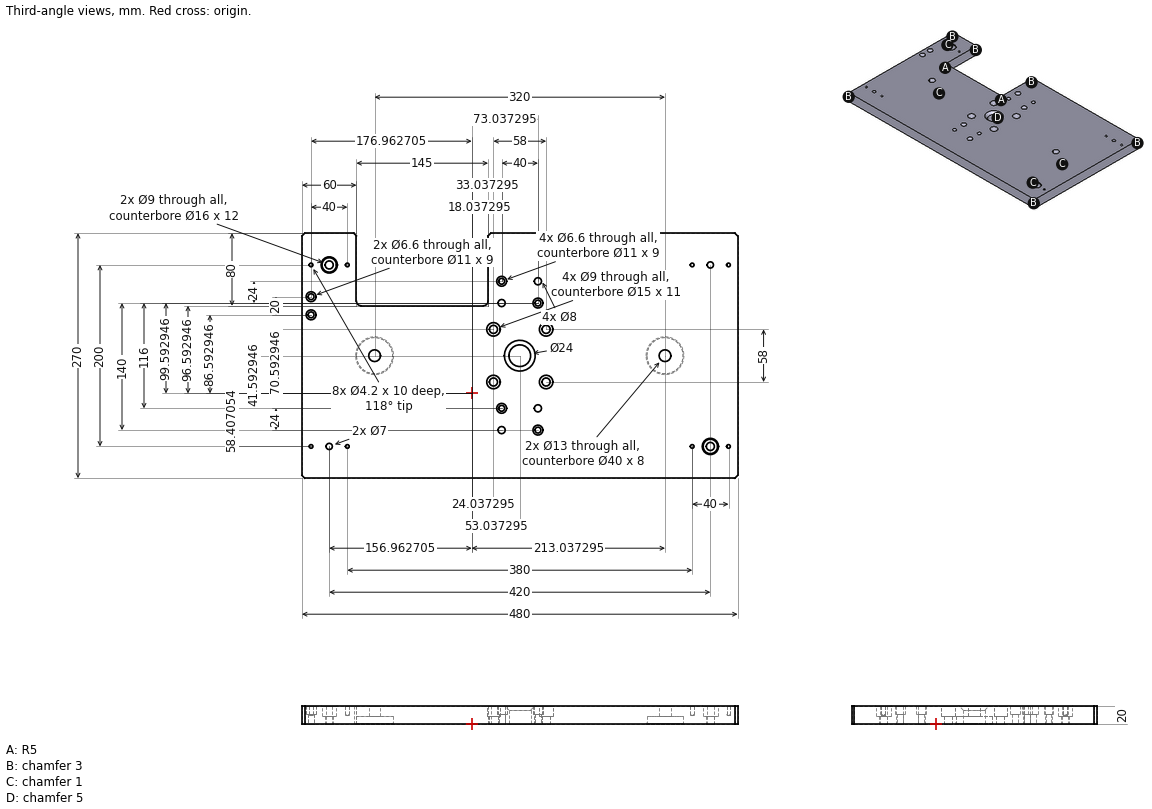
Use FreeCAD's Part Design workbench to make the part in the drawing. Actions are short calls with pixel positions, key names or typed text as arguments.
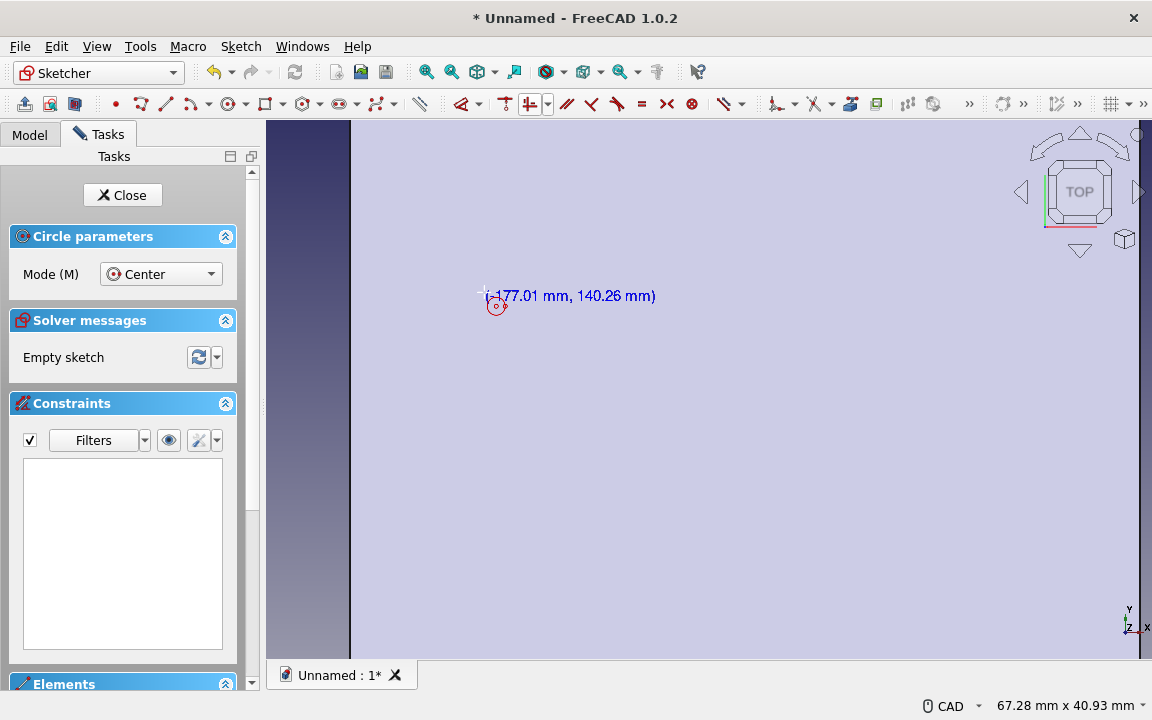
scroll(410, 292, down, 13)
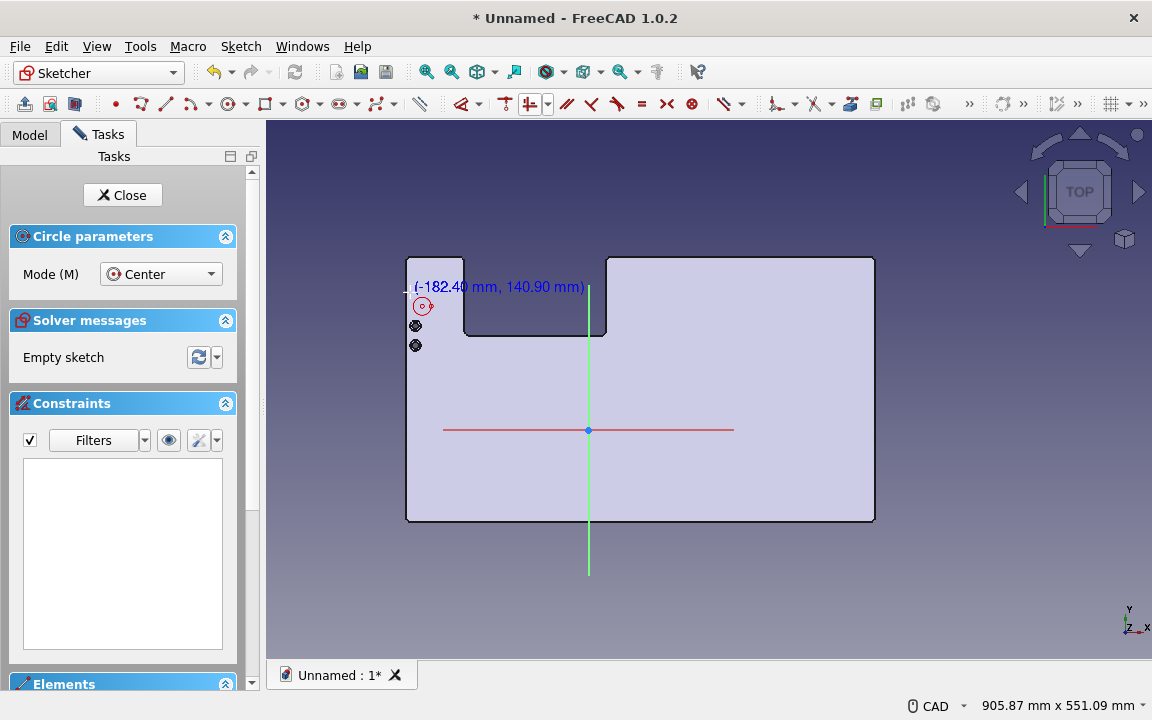
click(415, 292)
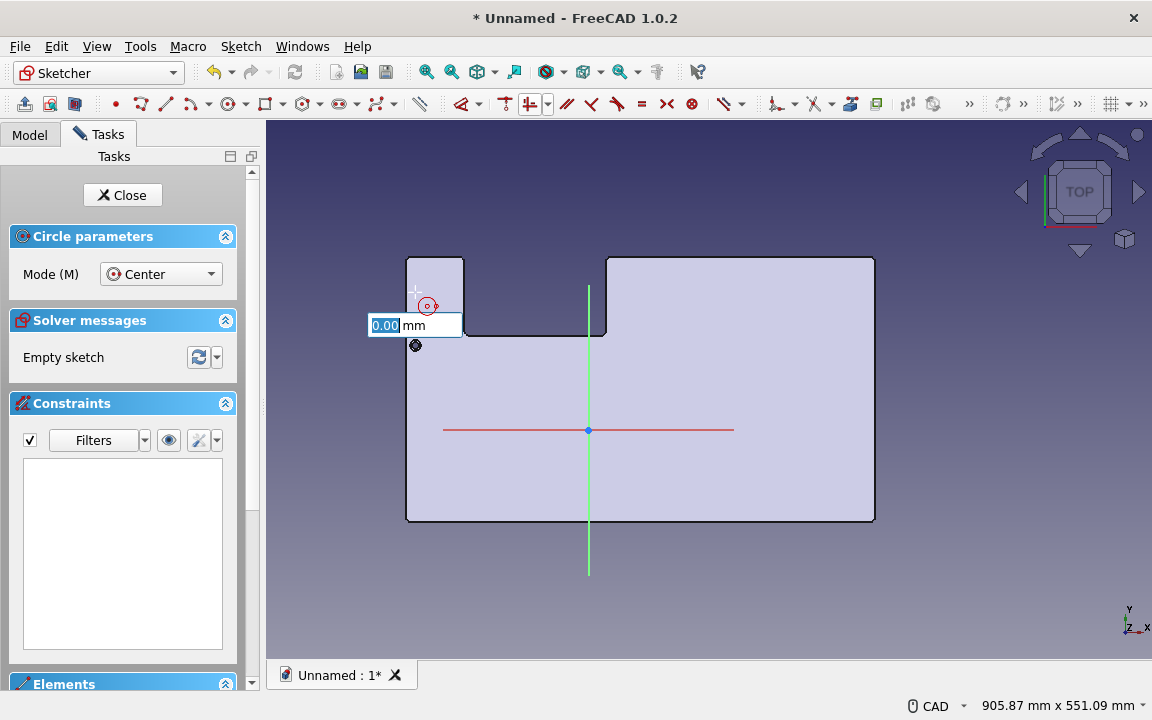
scroll(417, 290, up, 11)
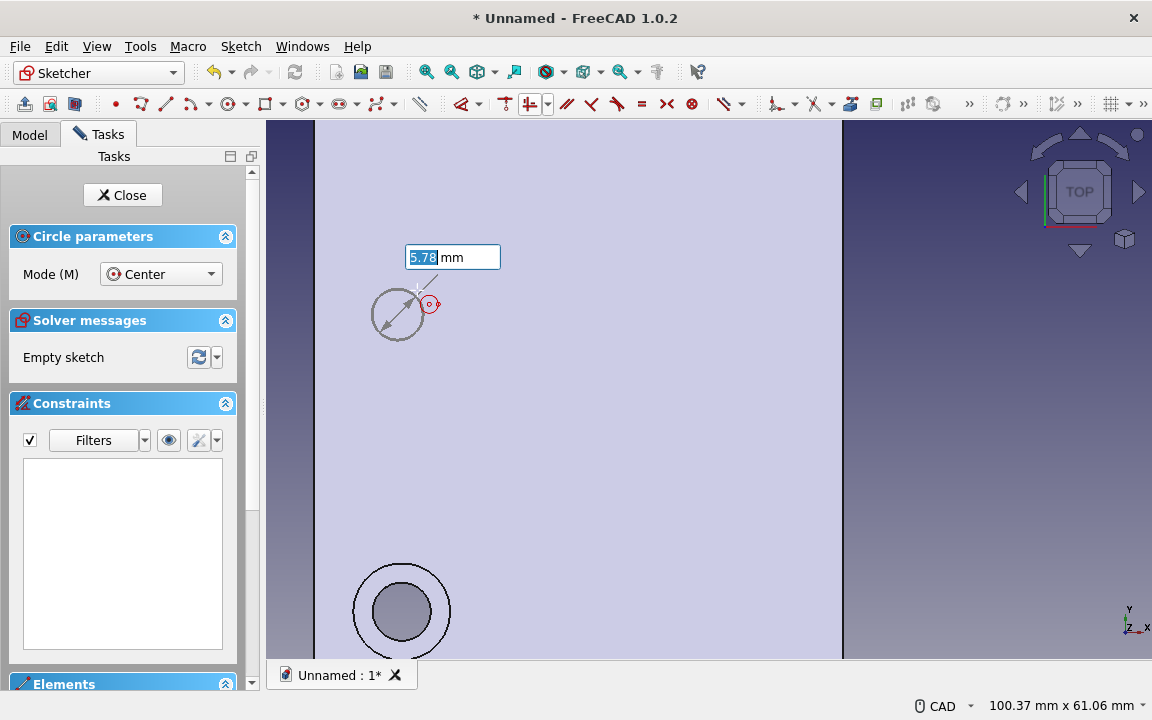
click(415, 290)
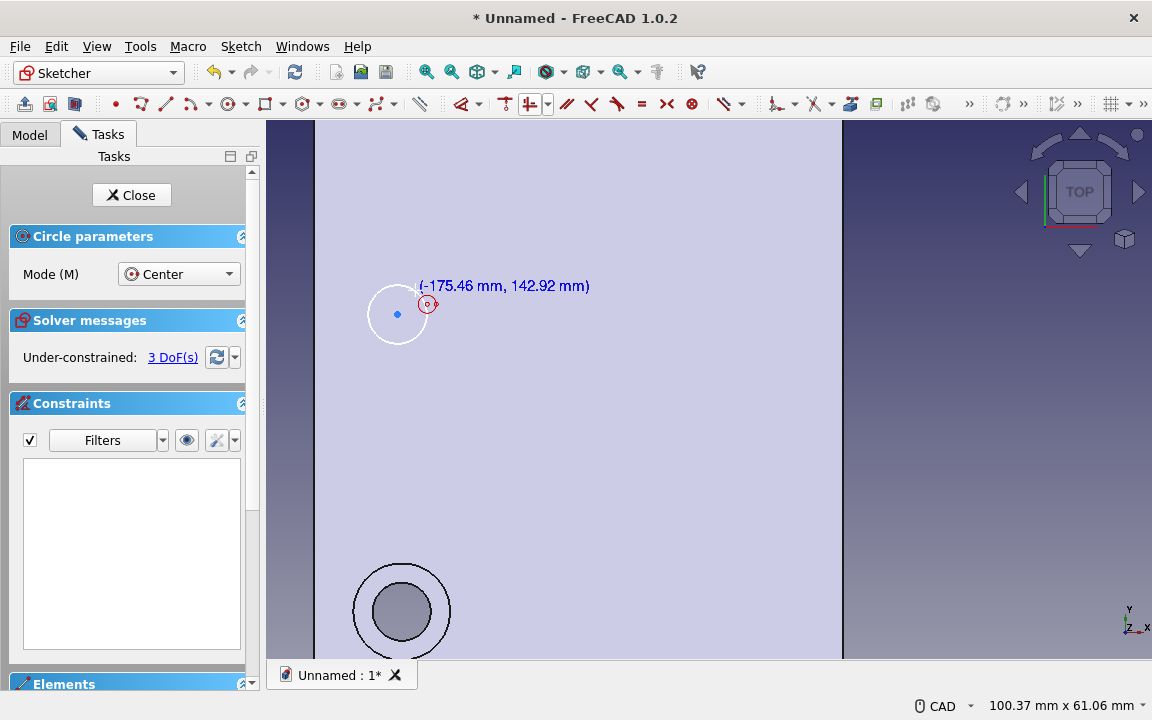
scroll(755, 303, up, 2)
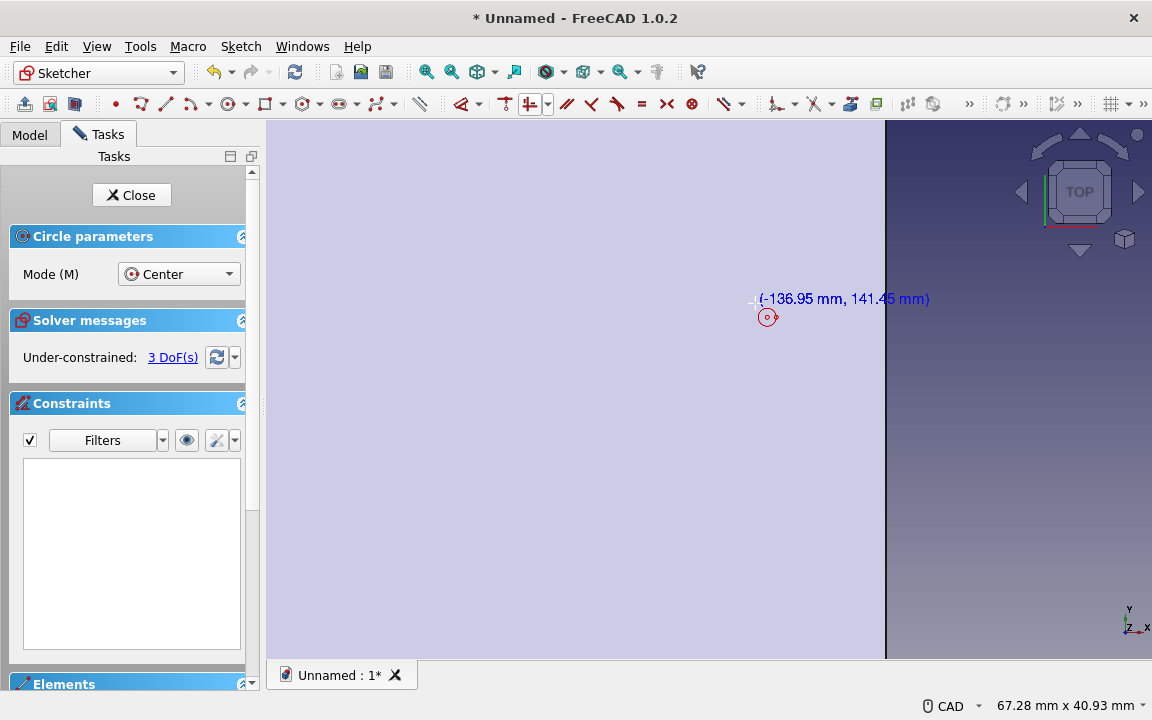
scroll(431, 291, down, 13)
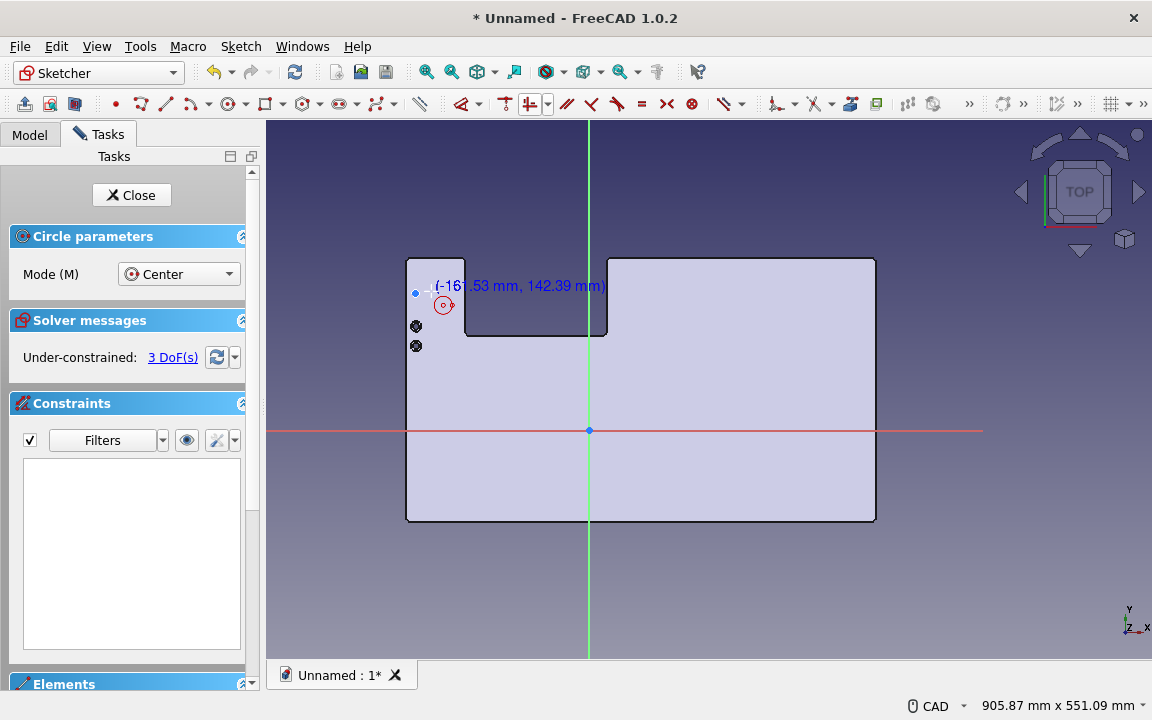
click(455, 292)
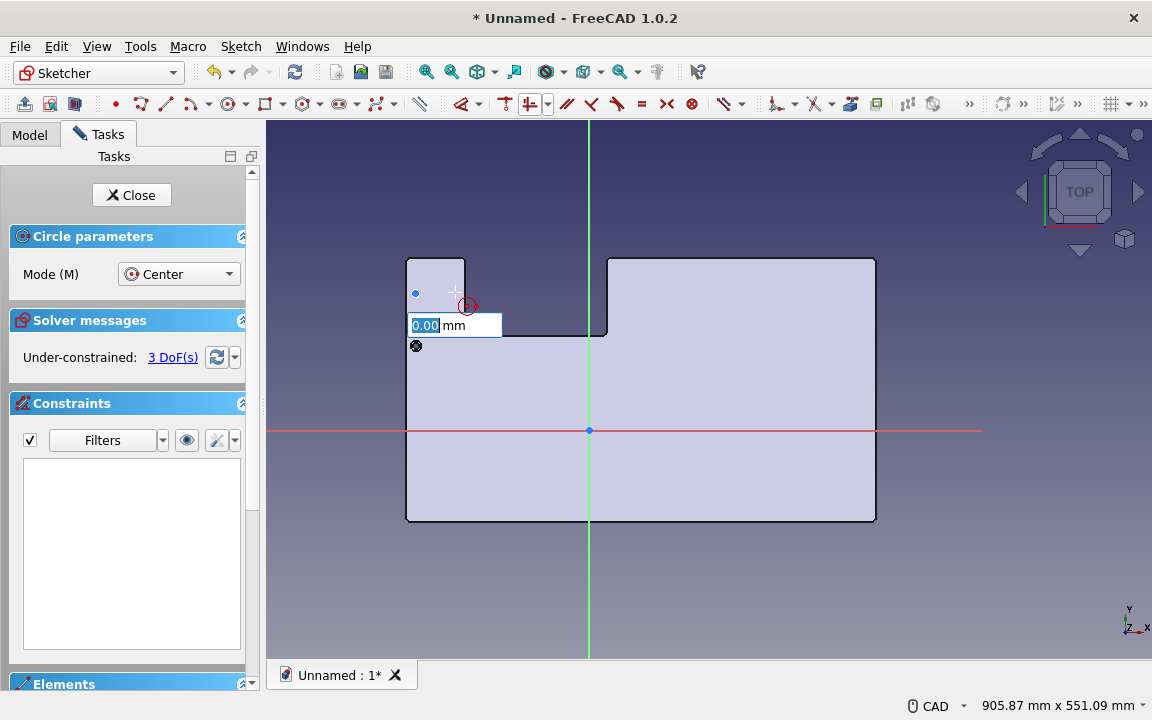
scroll(457, 291, up, 11)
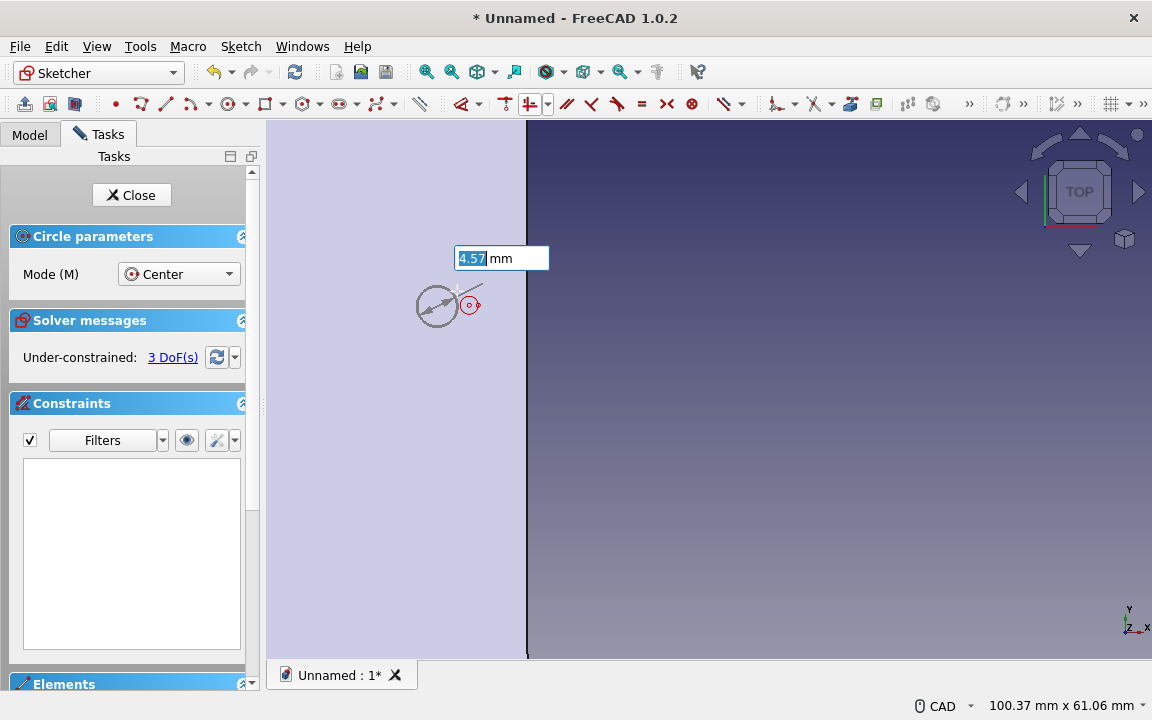
click(452, 286)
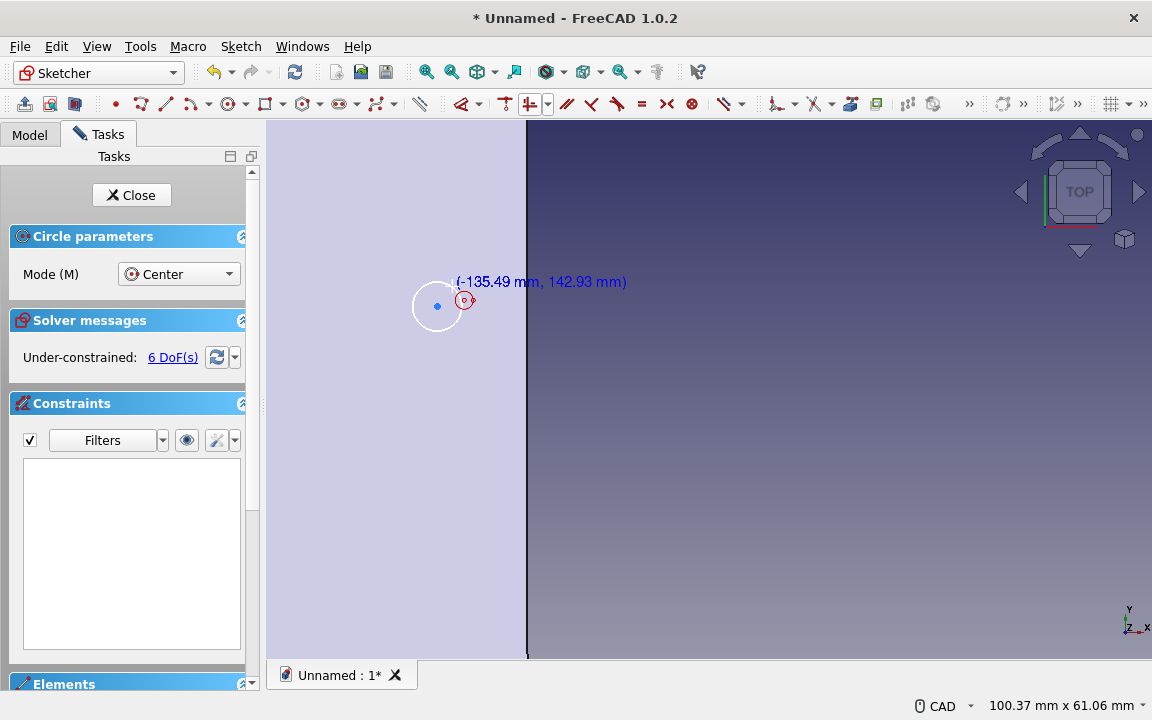
scroll(457, 291, down, 11)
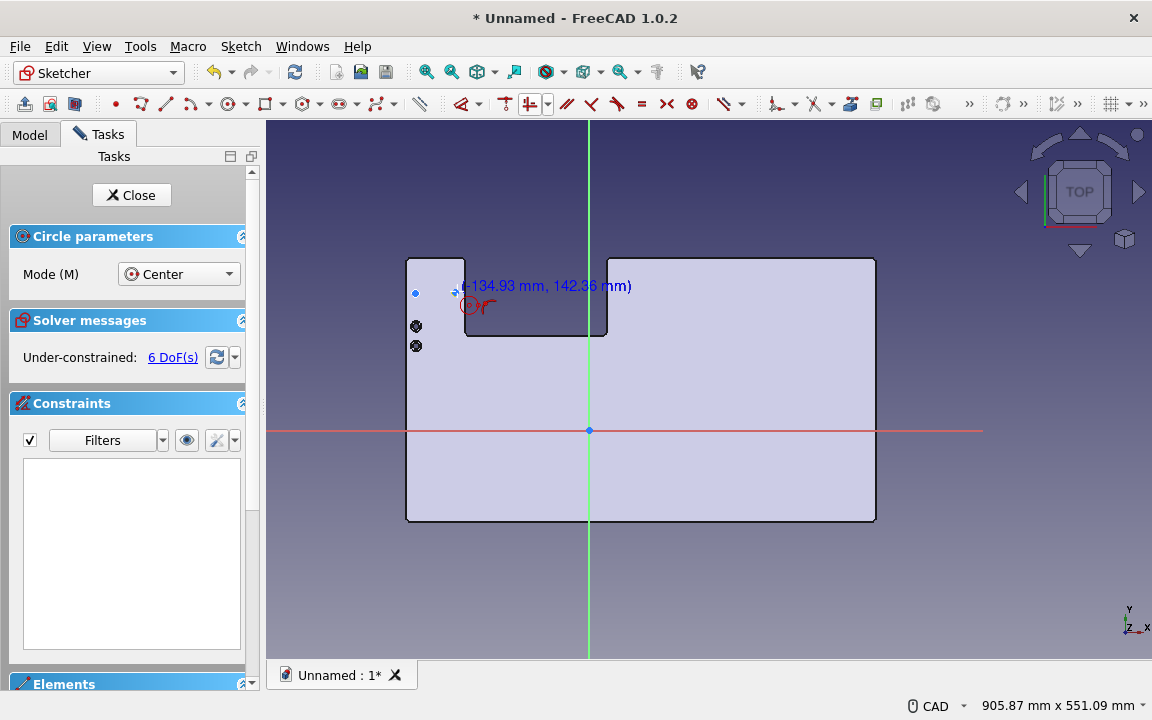
scroll(416, 488, up, 13)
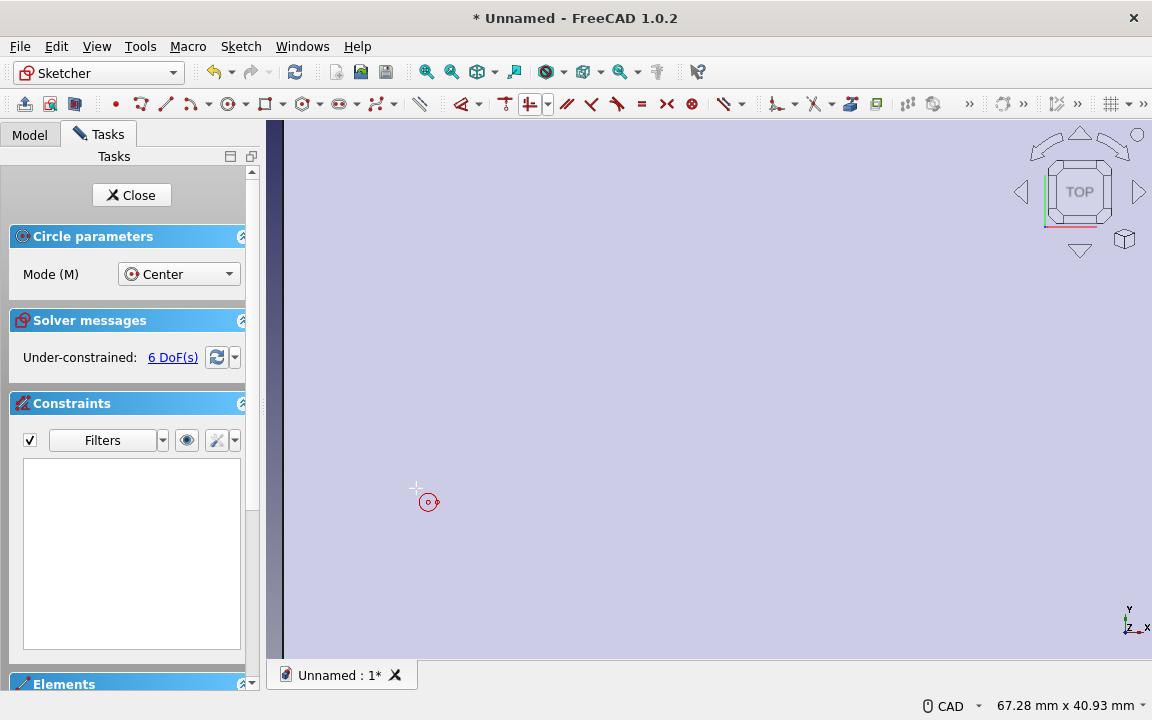
scroll(416, 488, down, 13)